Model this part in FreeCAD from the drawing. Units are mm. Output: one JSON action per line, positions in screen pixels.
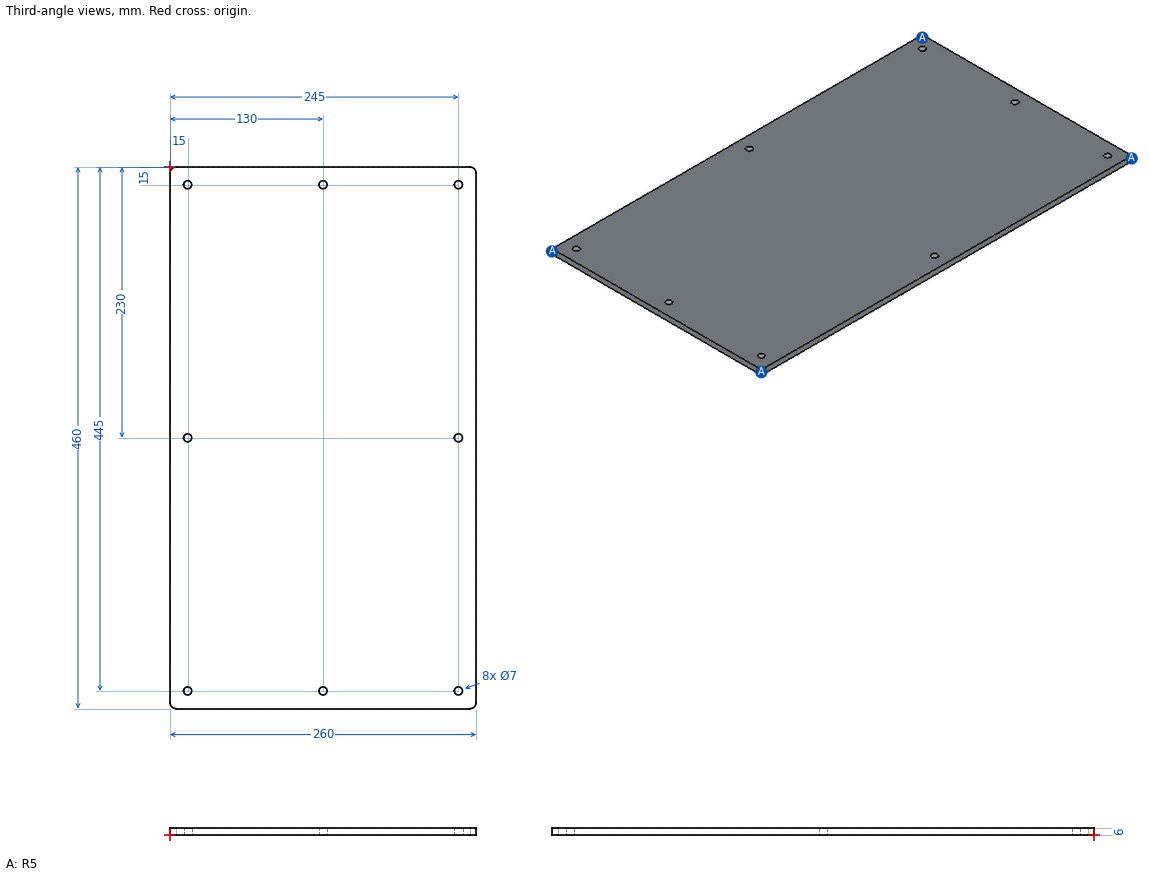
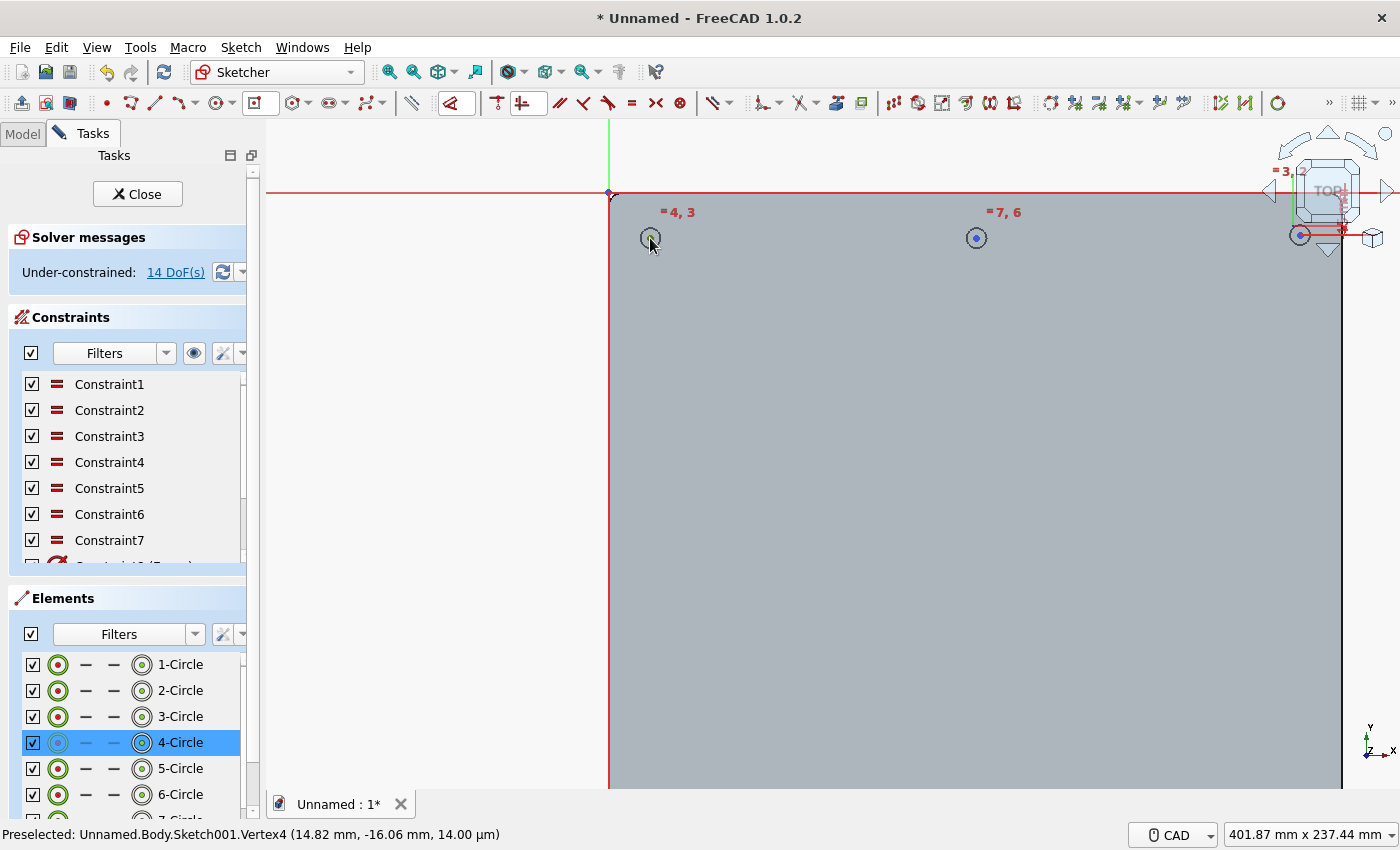
{"action": "key", "text": "l"}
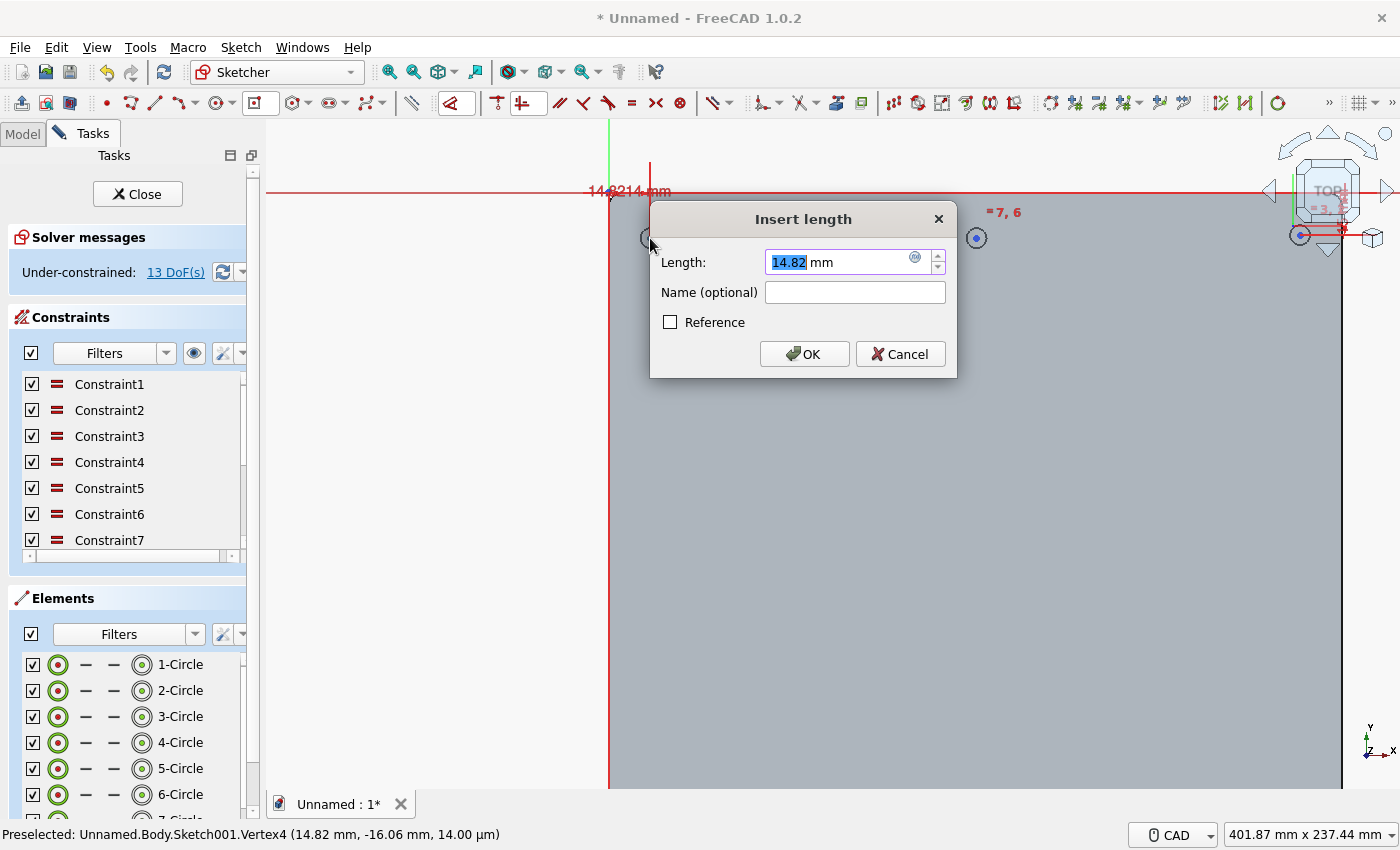
{"action": "type", "text": "15"}
{"action": "key", "text": "Return"}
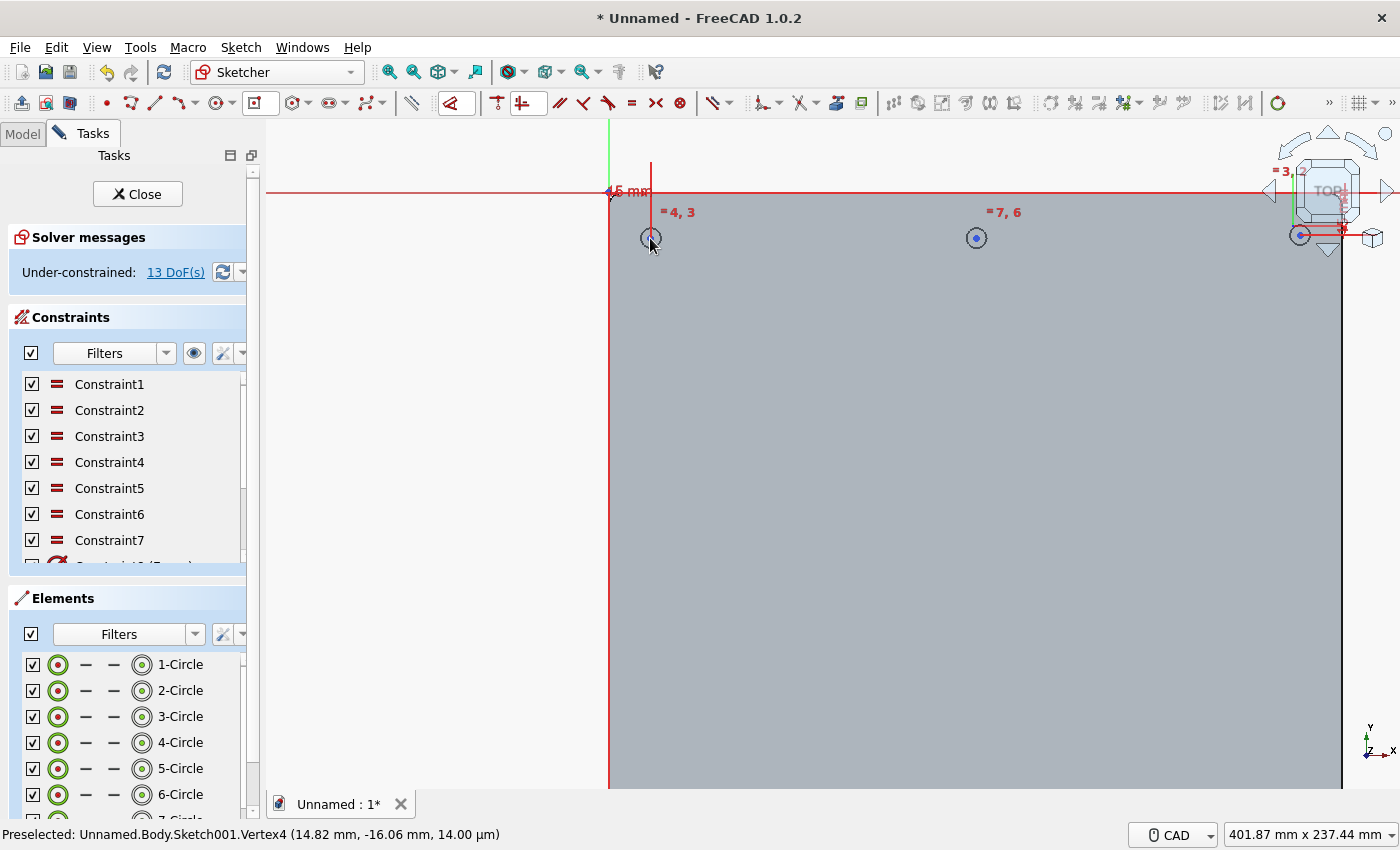
{"action": "left_click", "coordinate": [651, 238]}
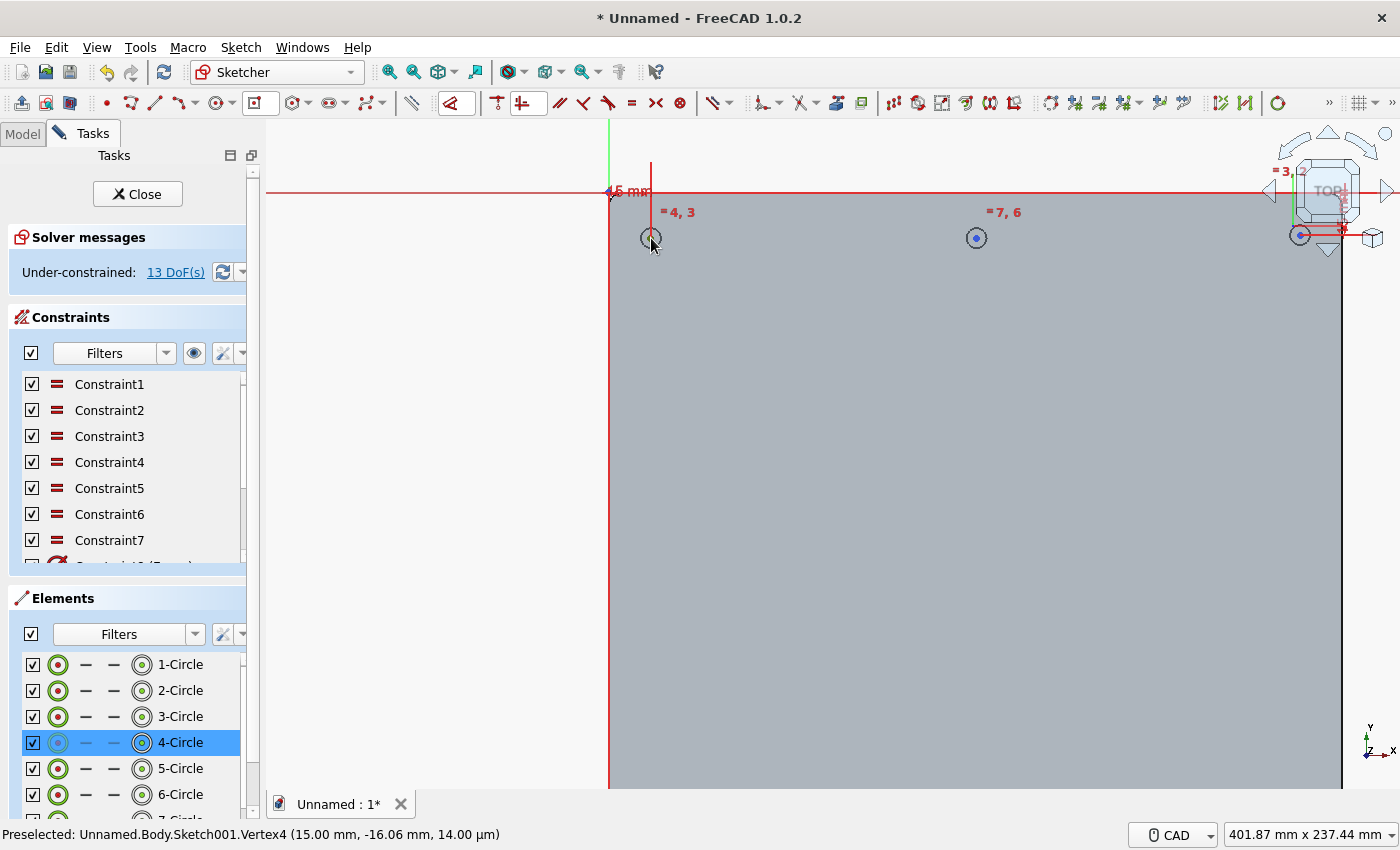
{"action": "left_click", "coordinate": [470, 104]}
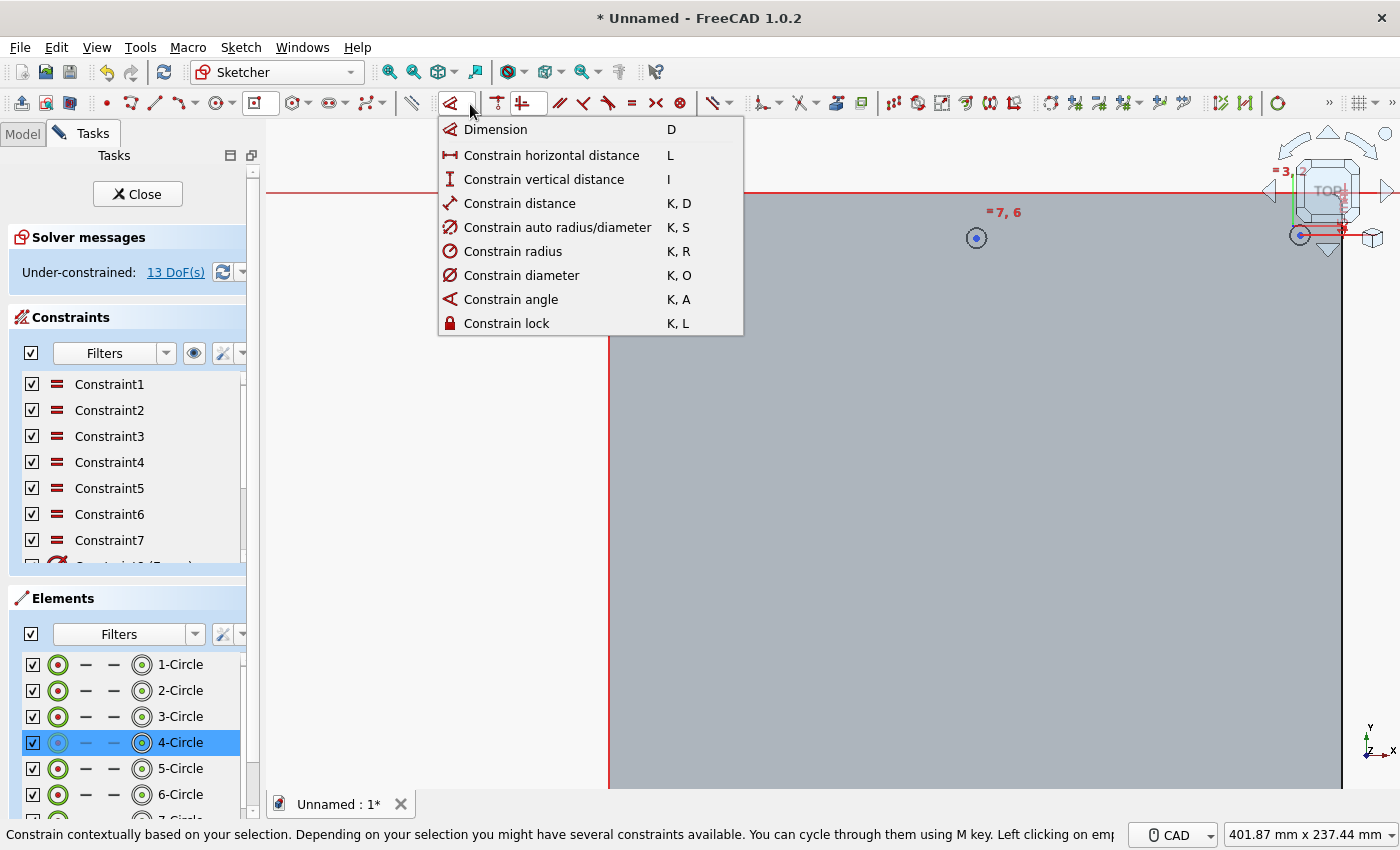
{"action": "left_click", "coordinate": [591, 179]}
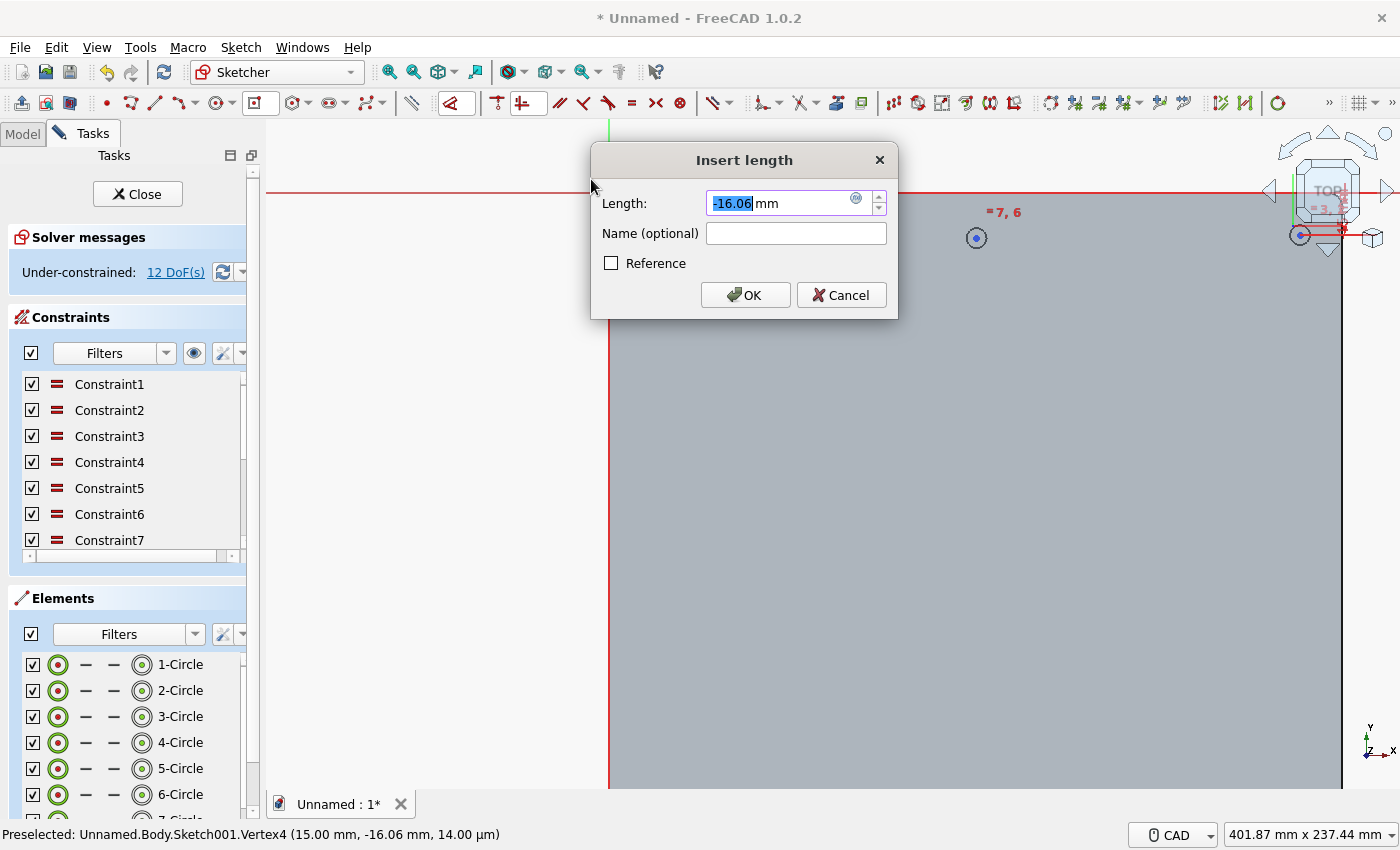
{"action": "type", "text": "-15"}
{"action": "key", "text": "Return"}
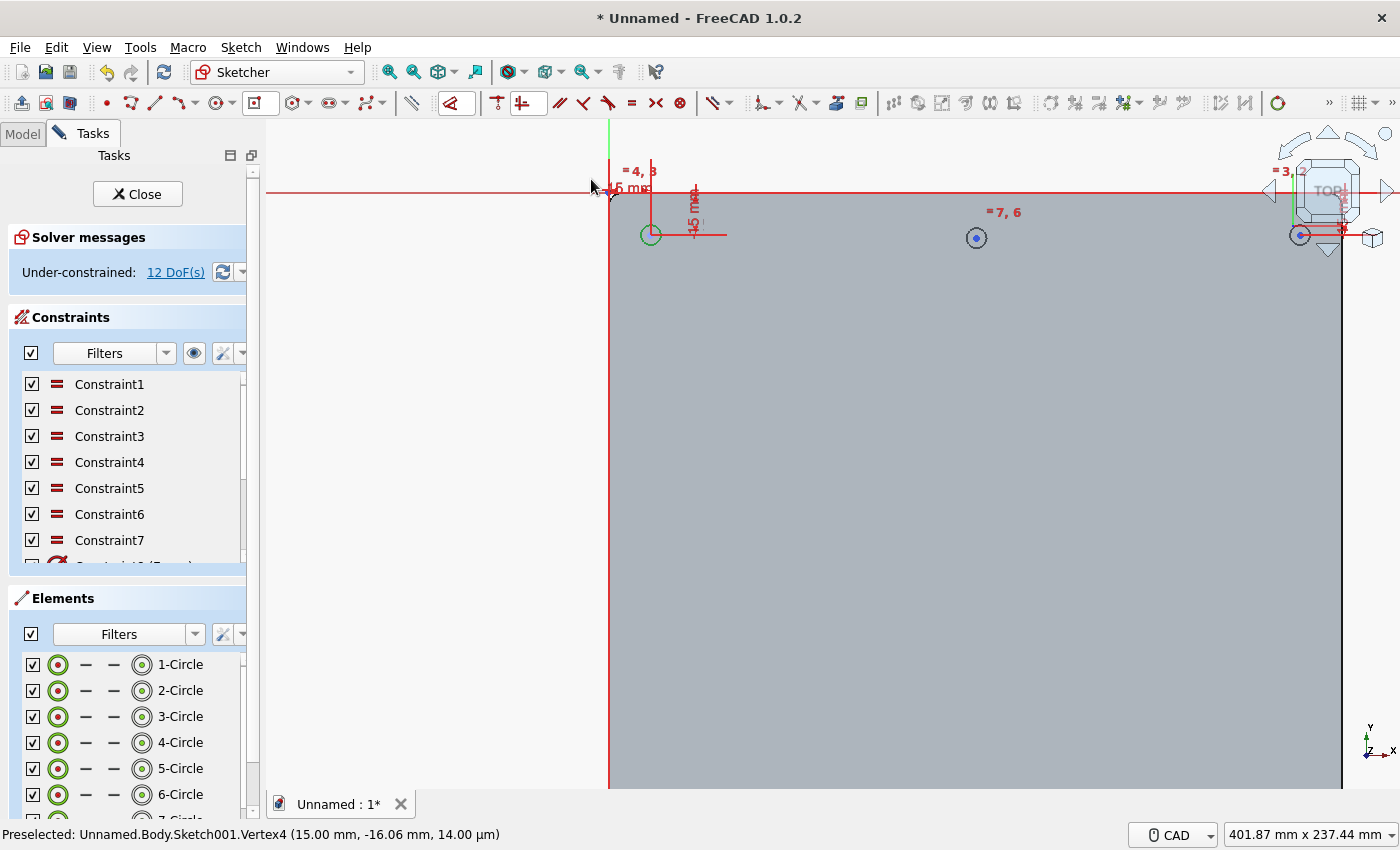
{"action": "left_click", "coordinate": [977, 238]}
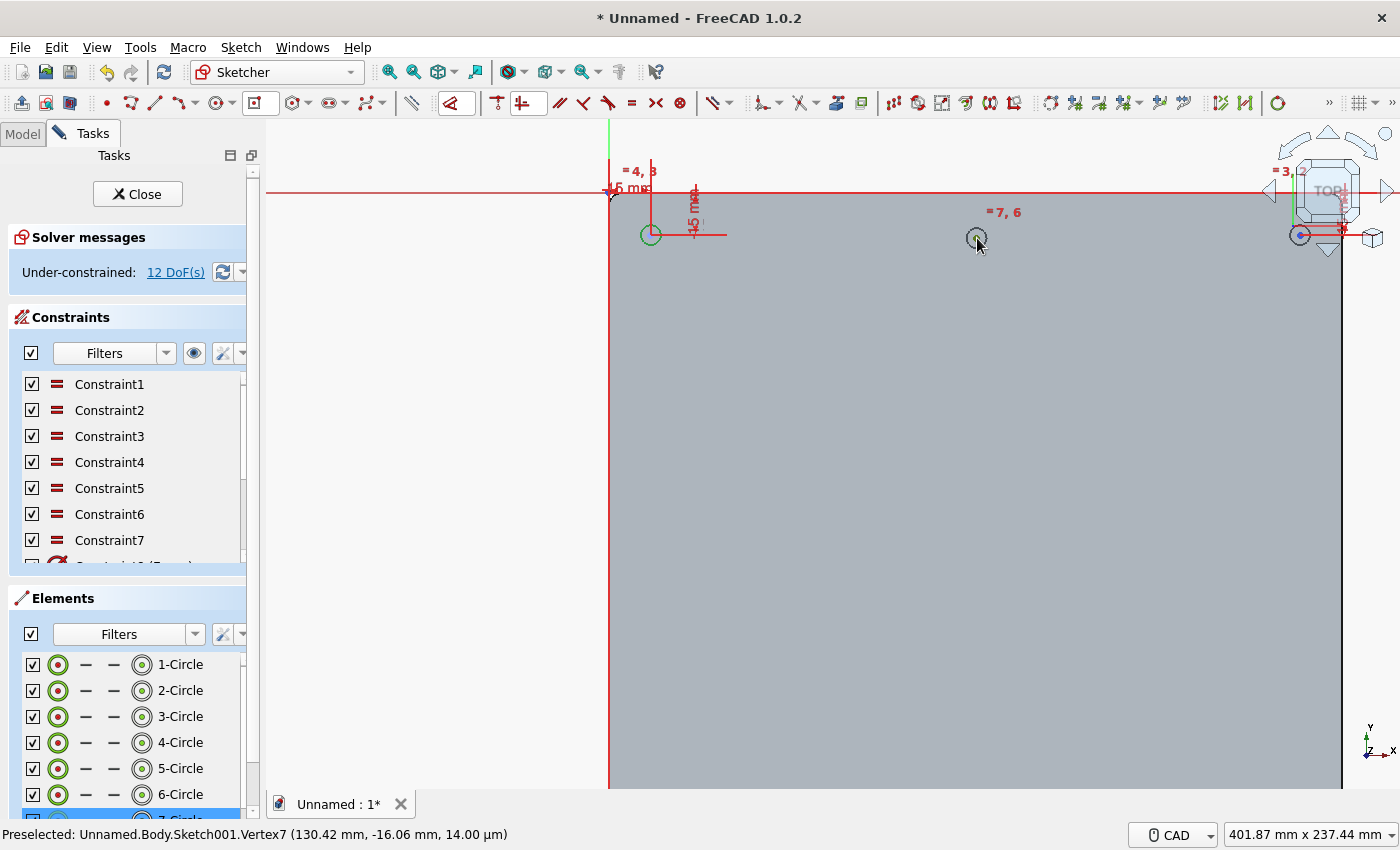
{"action": "key", "text": "i"}